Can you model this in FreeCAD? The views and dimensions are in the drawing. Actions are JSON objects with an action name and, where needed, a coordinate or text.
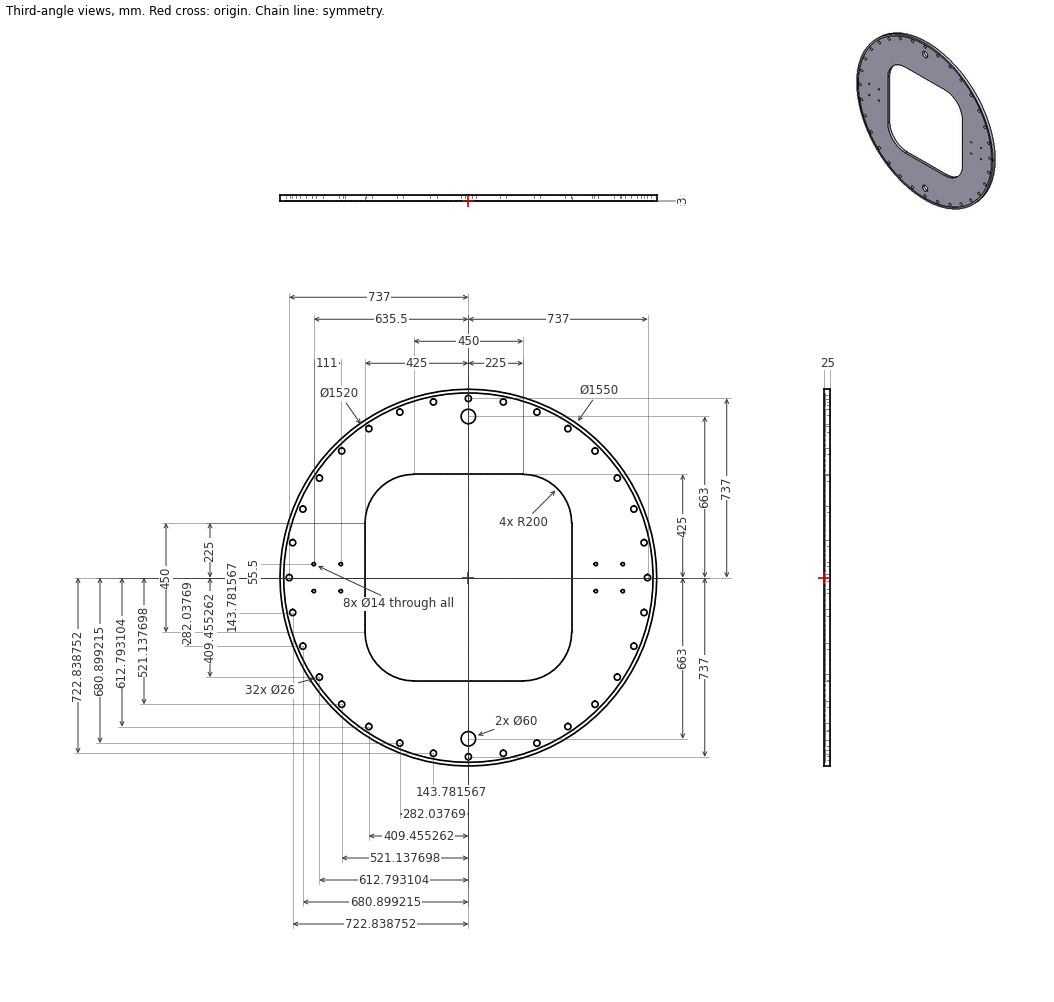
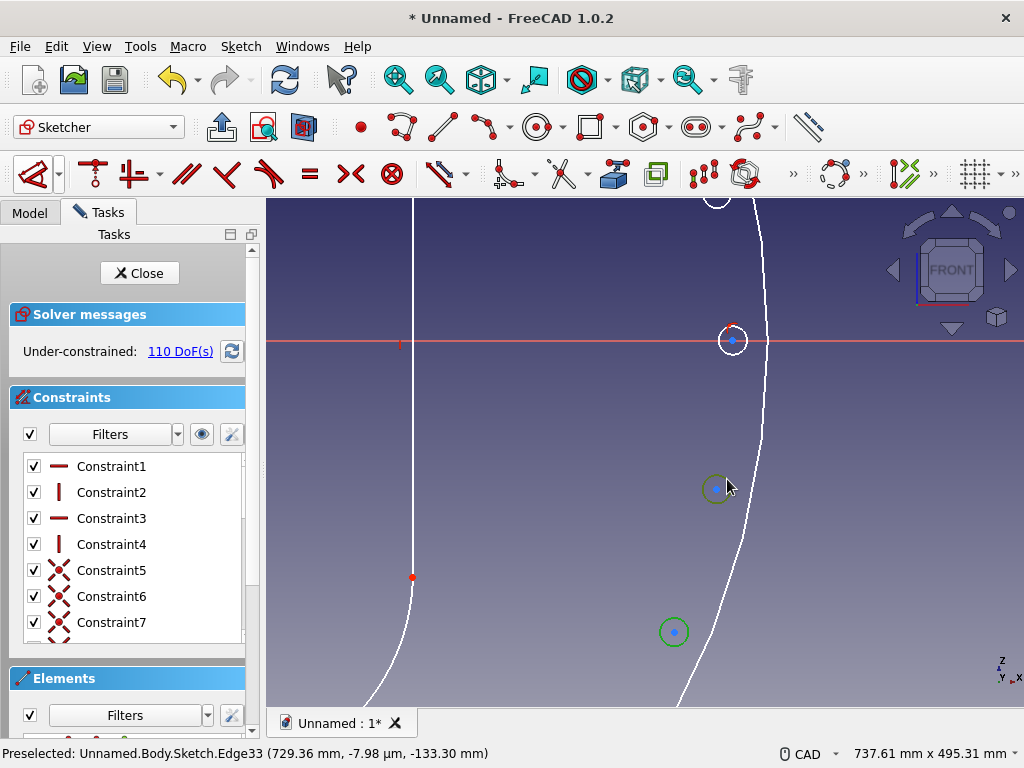
{"action": "scroll", "coordinate": [743, 330], "scroll_direction": "up", "scroll_amount": 2}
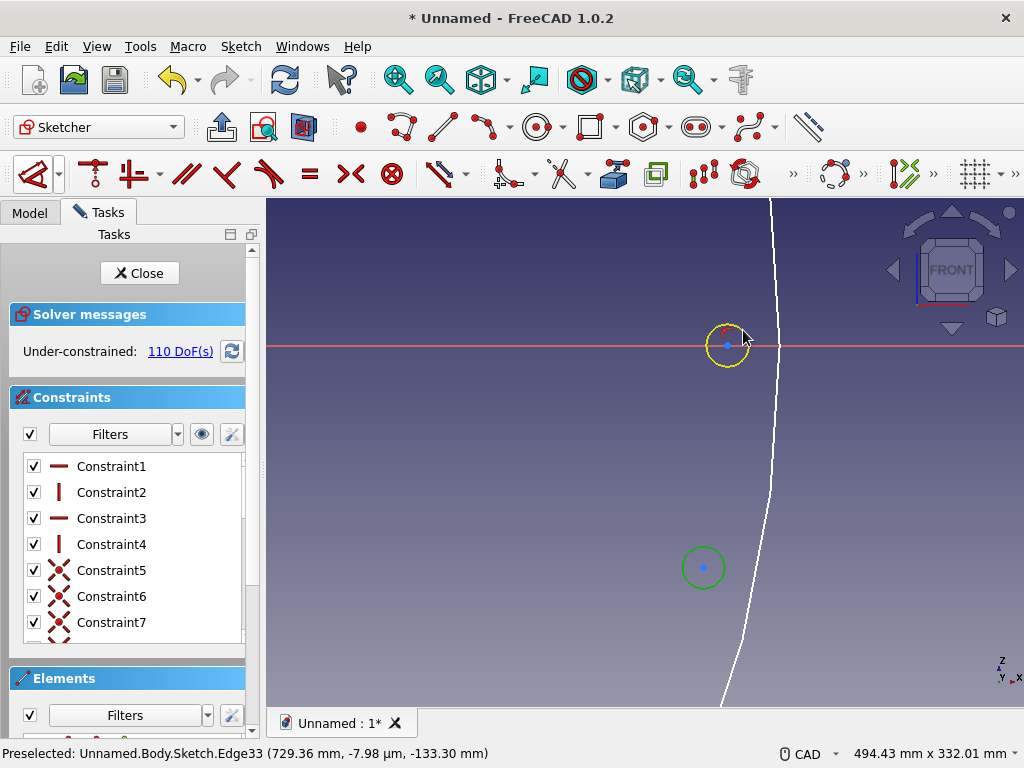
{"action": "left_click", "coordinate": [743, 331]}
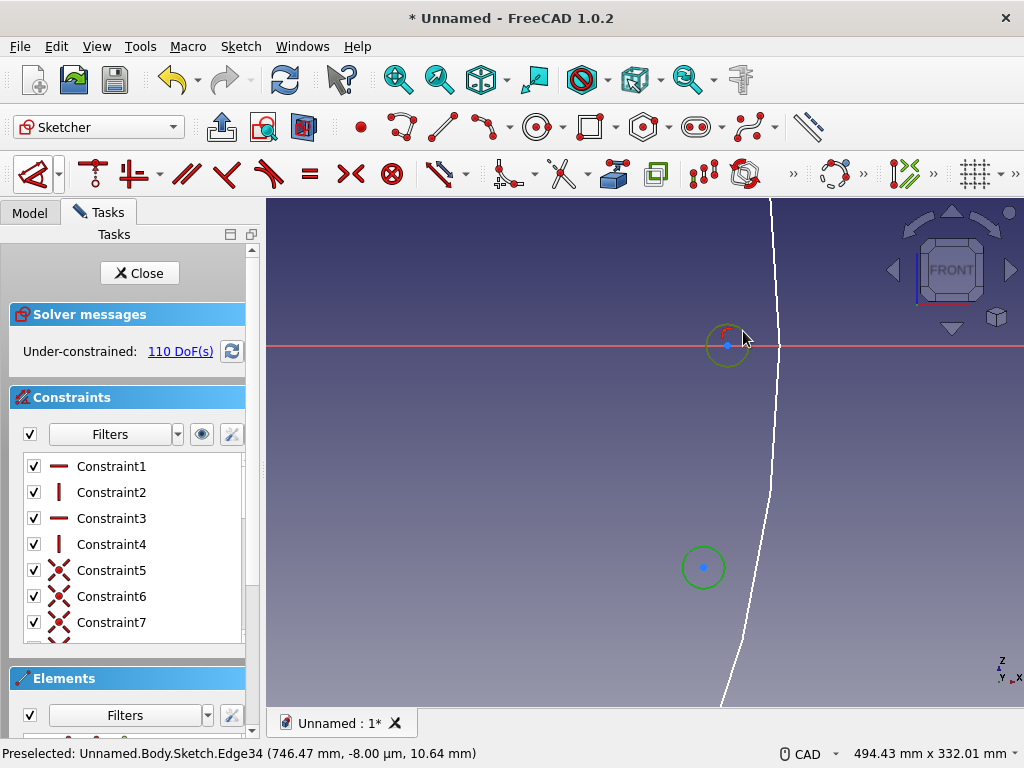
{"action": "scroll", "coordinate": [730, 469], "scroll_direction": "down", "scroll_amount": 10}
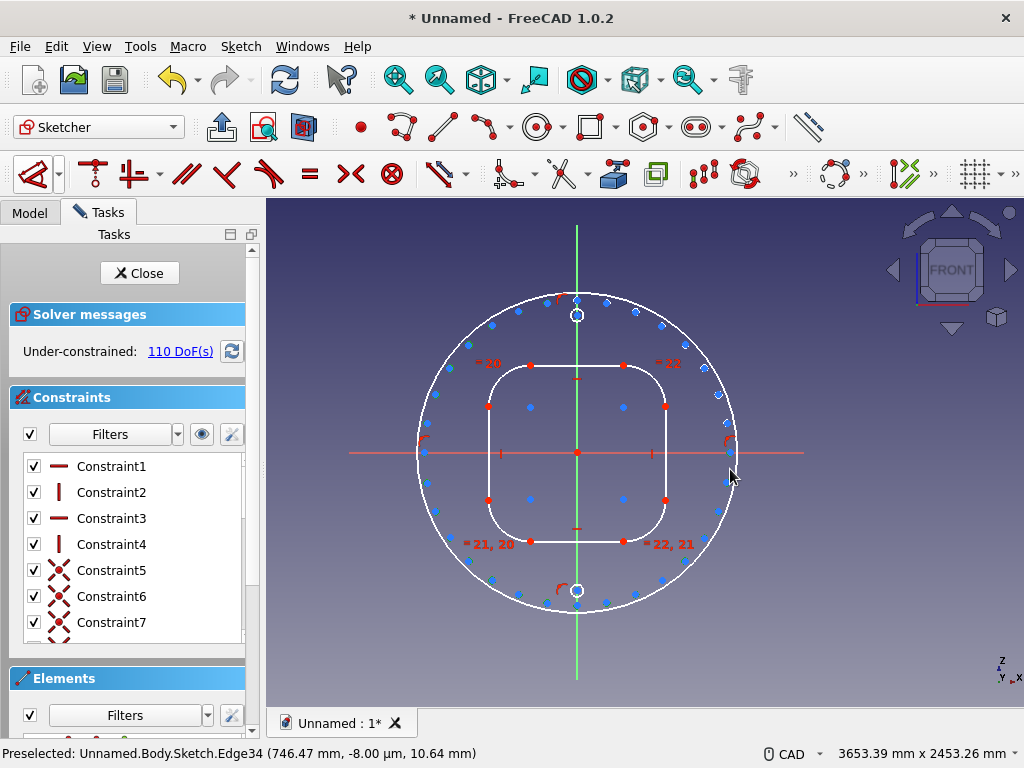
{"action": "scroll", "coordinate": [579, 298], "scroll_direction": "up", "scroll_amount": 10}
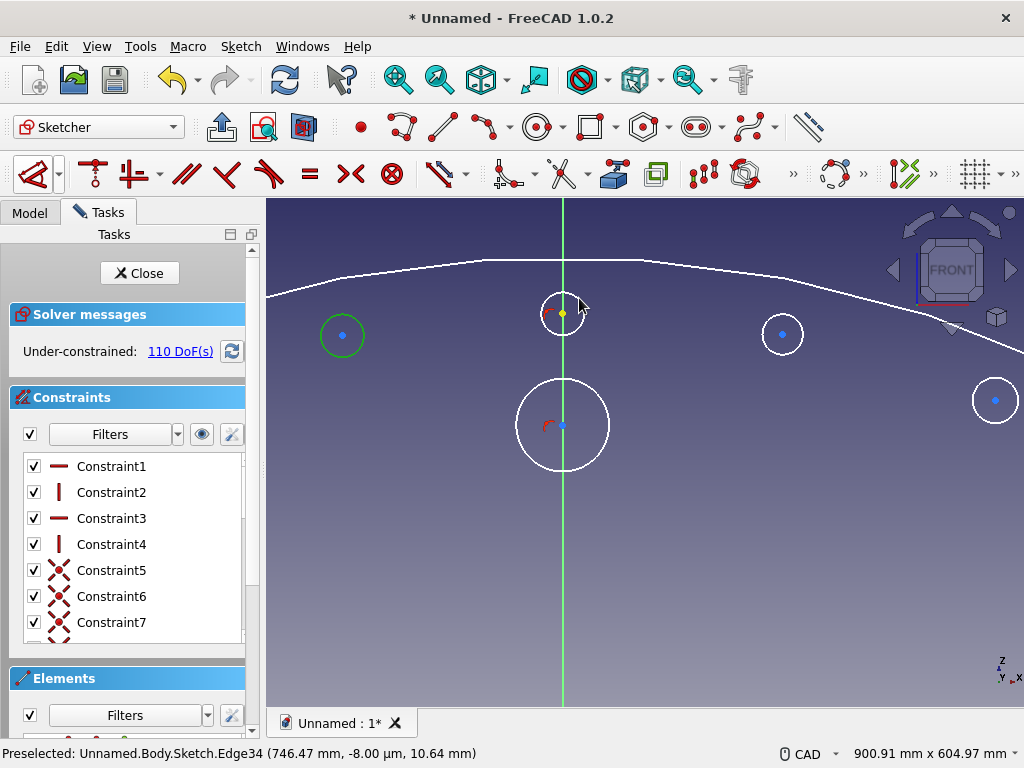
{"action": "left_click", "coordinate": [578, 299]}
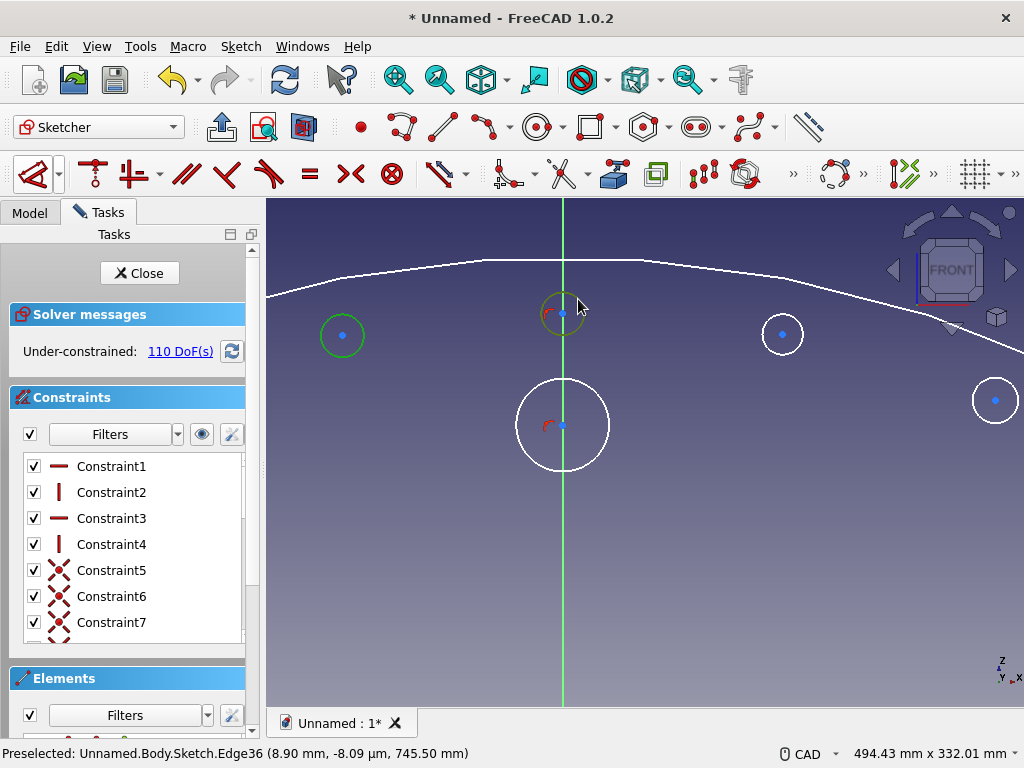
{"action": "left_click", "coordinate": [797, 320]}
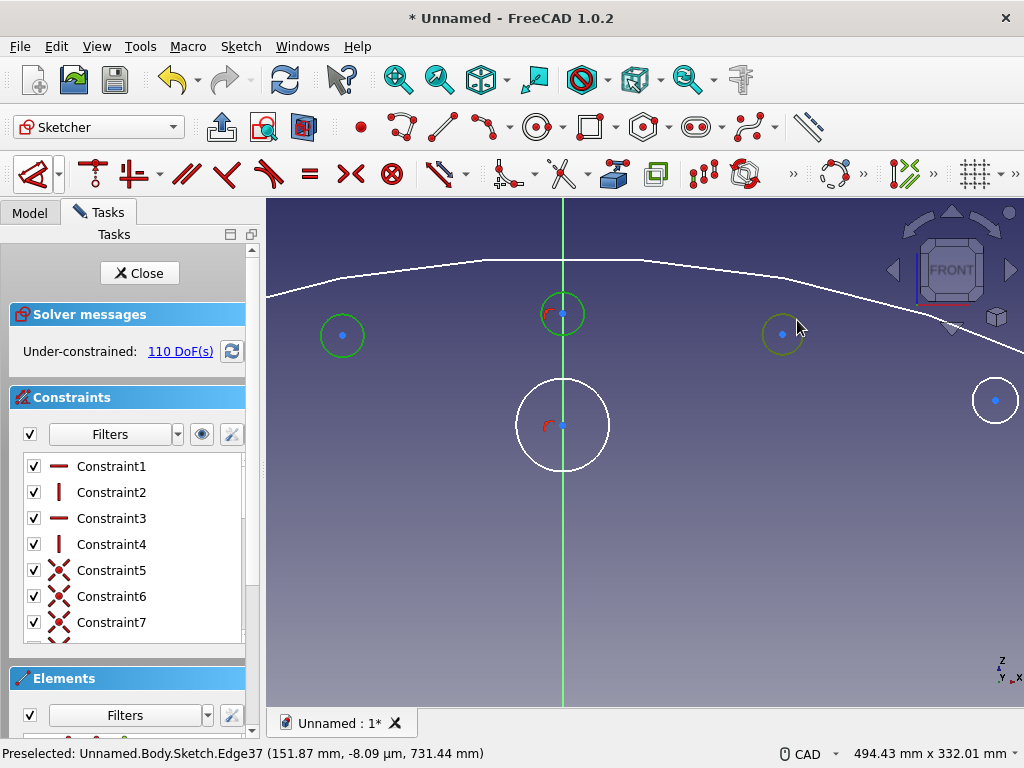
{"action": "scroll", "coordinate": [579, 298], "scroll_direction": "down", "scroll_amount": 10}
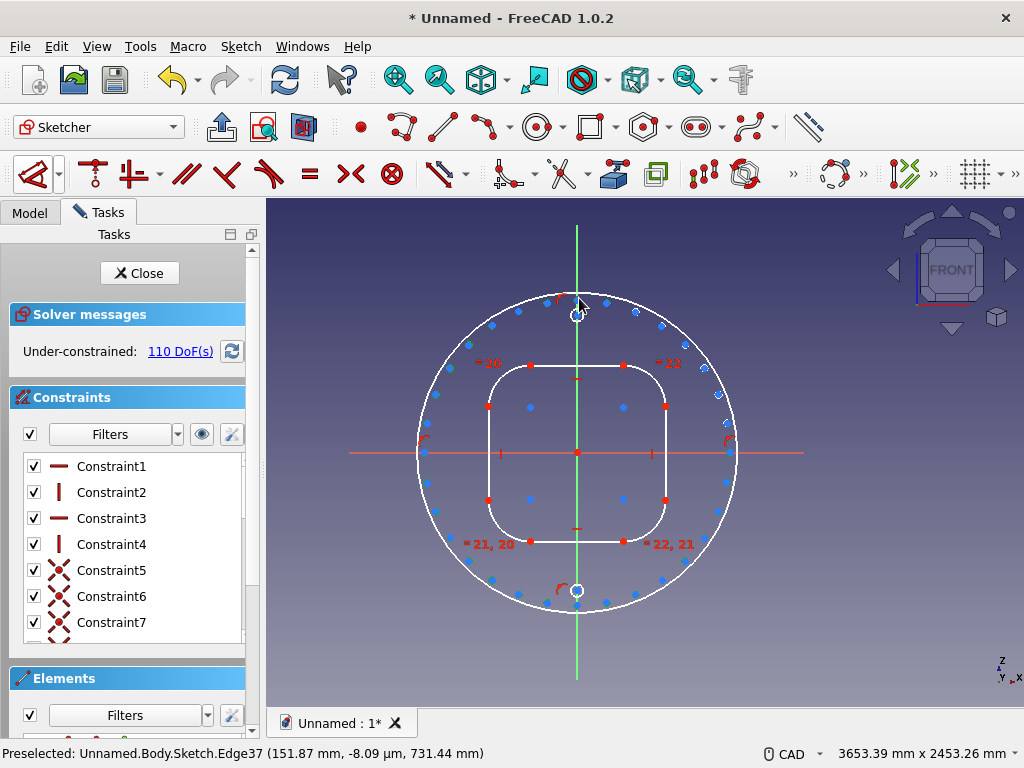
{"action": "scroll", "coordinate": [638, 310], "scroll_direction": "up", "scroll_amount": 8}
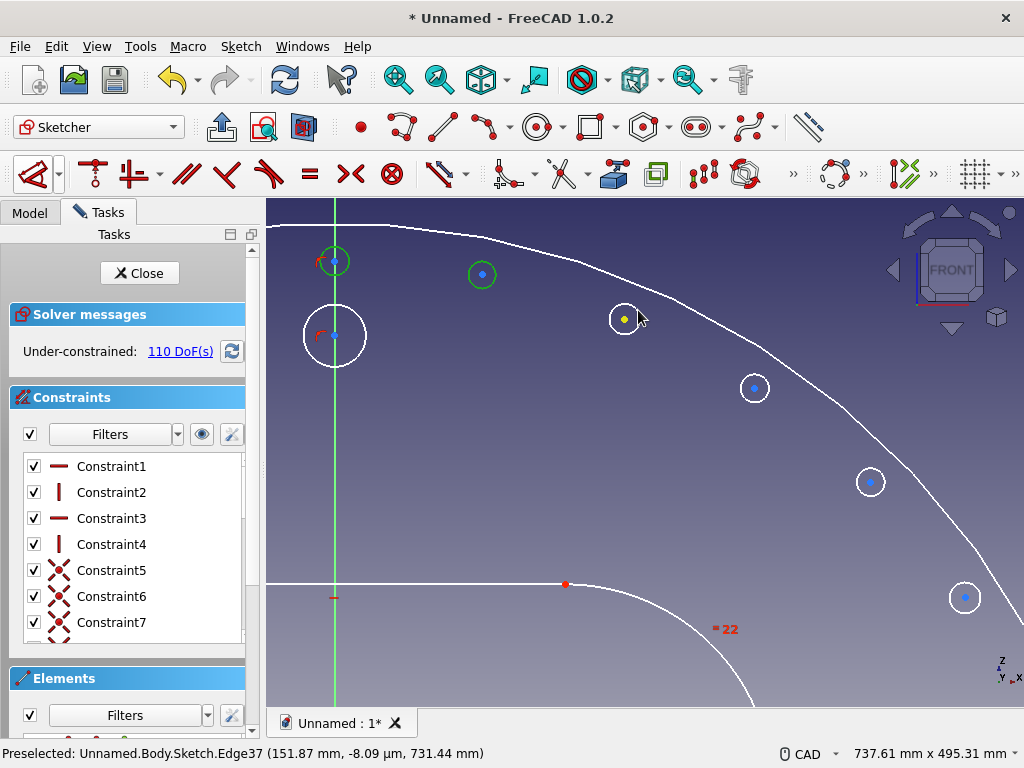
{"action": "left_click", "coordinate": [636, 308]}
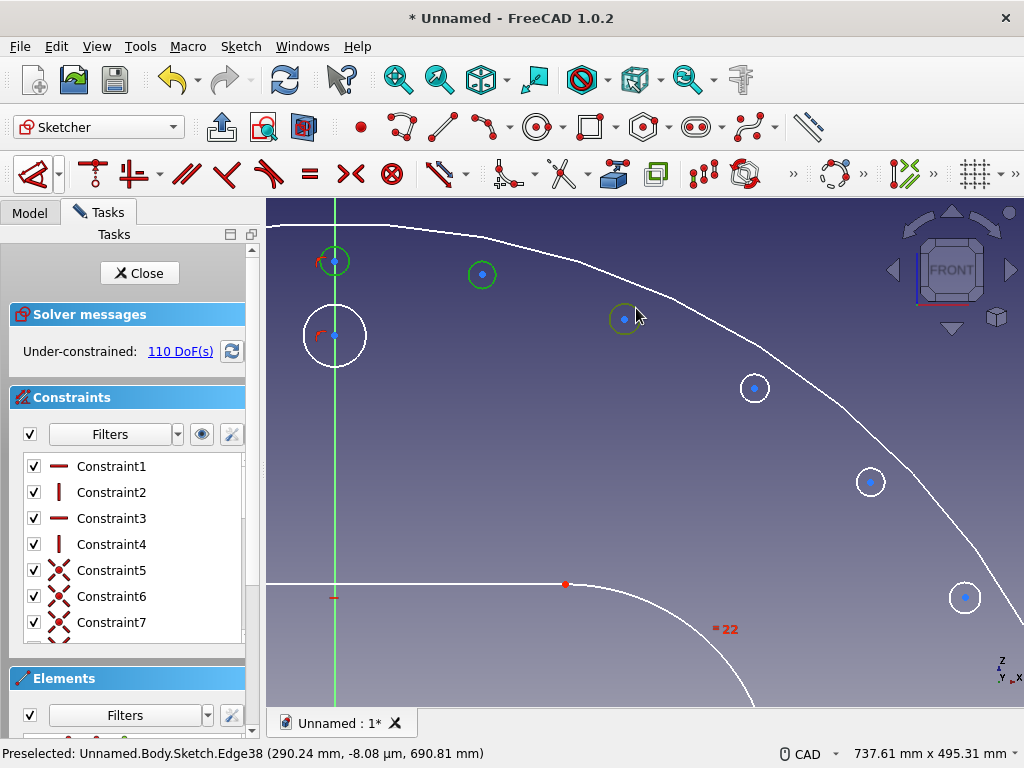
{"action": "scroll", "coordinate": [638, 310], "scroll_direction": "down", "scroll_amount": 8}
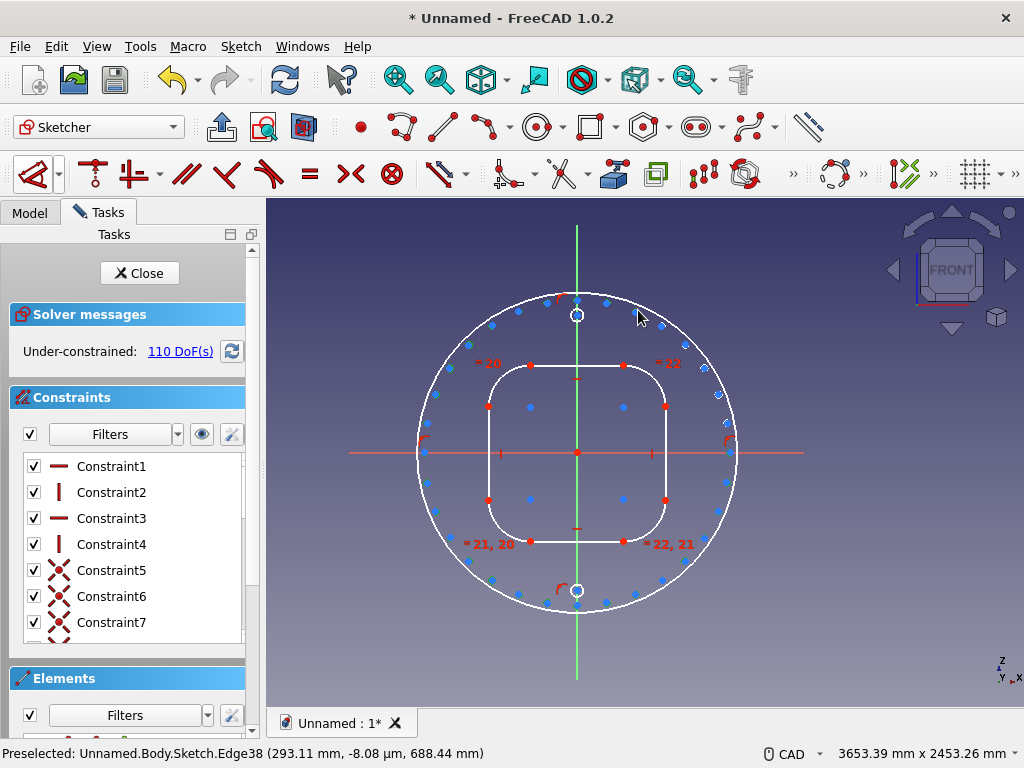
{"action": "scroll", "coordinate": [729, 421], "scroll_direction": "up", "scroll_amount": 9}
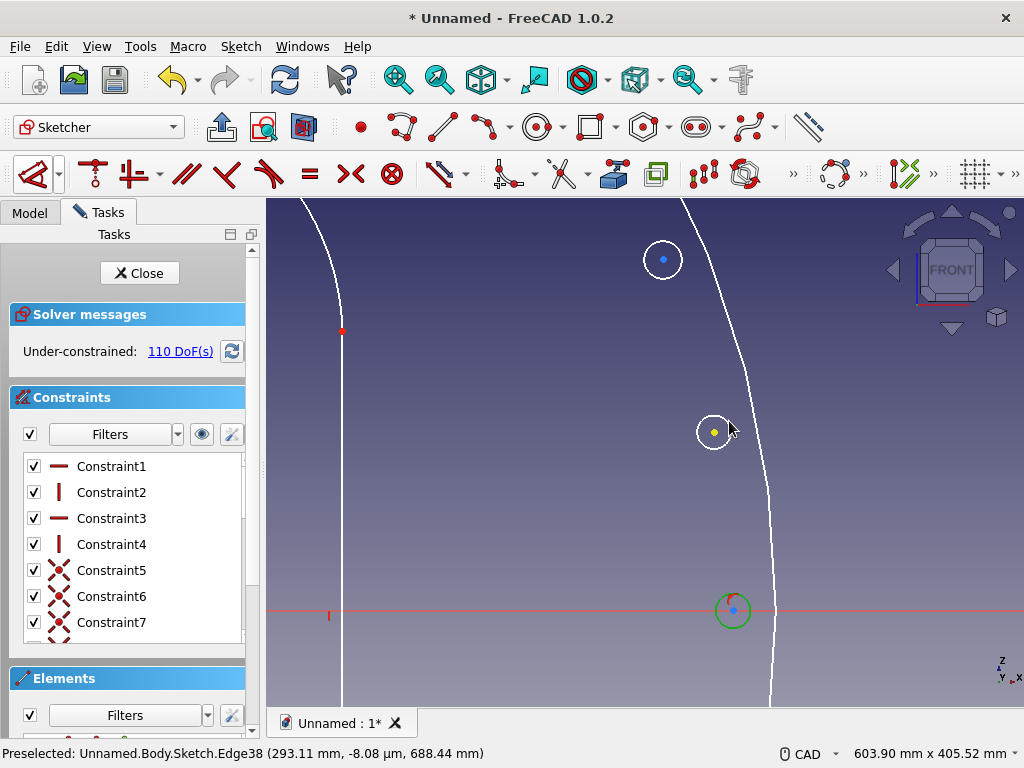
{"action": "left_click", "coordinate": [726, 420]}